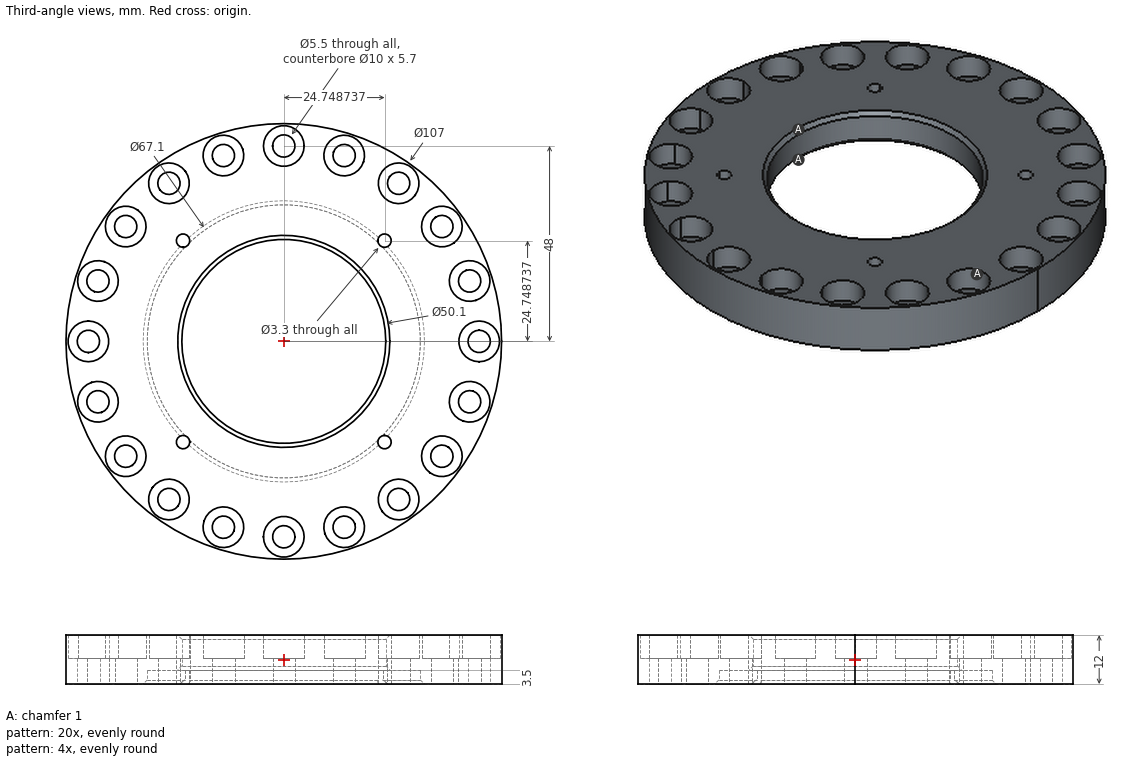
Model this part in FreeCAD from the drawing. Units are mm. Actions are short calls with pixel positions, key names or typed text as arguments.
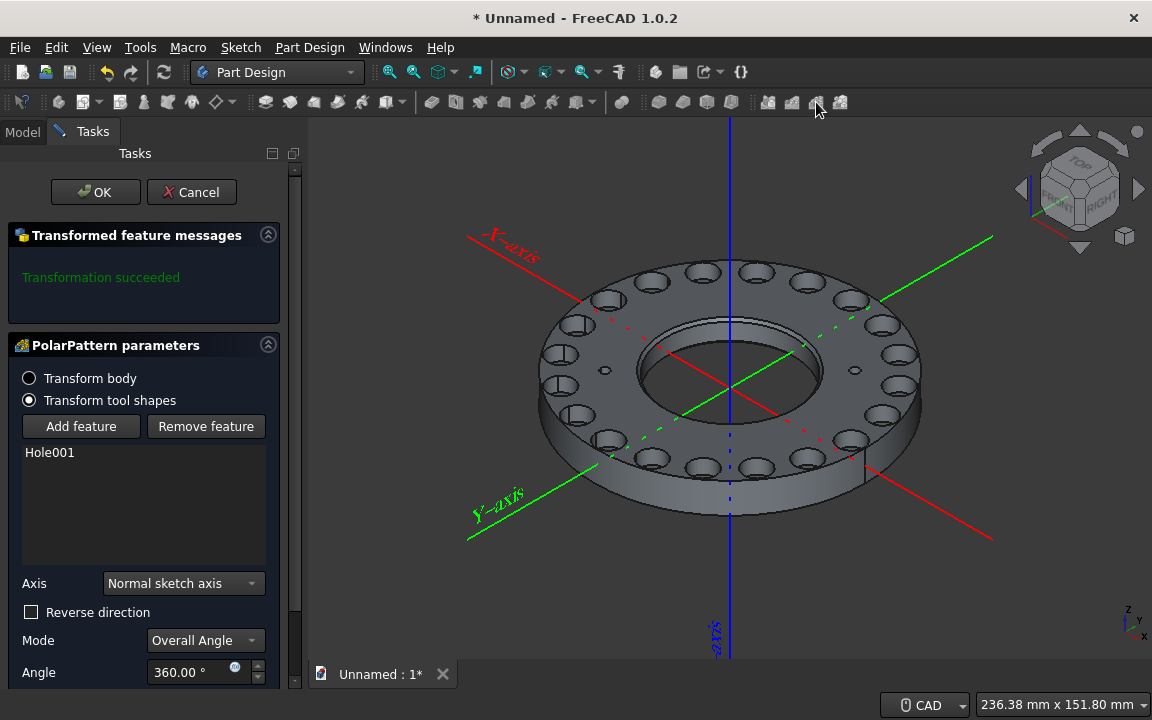
click(184, 584)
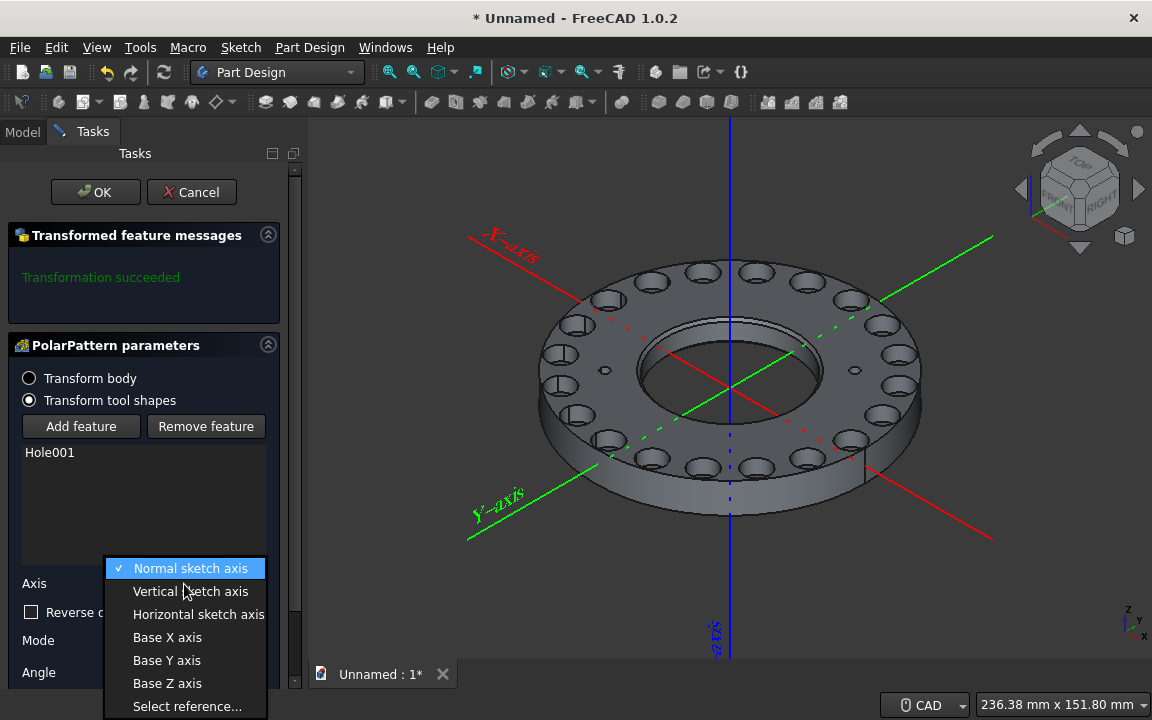
click(184, 684)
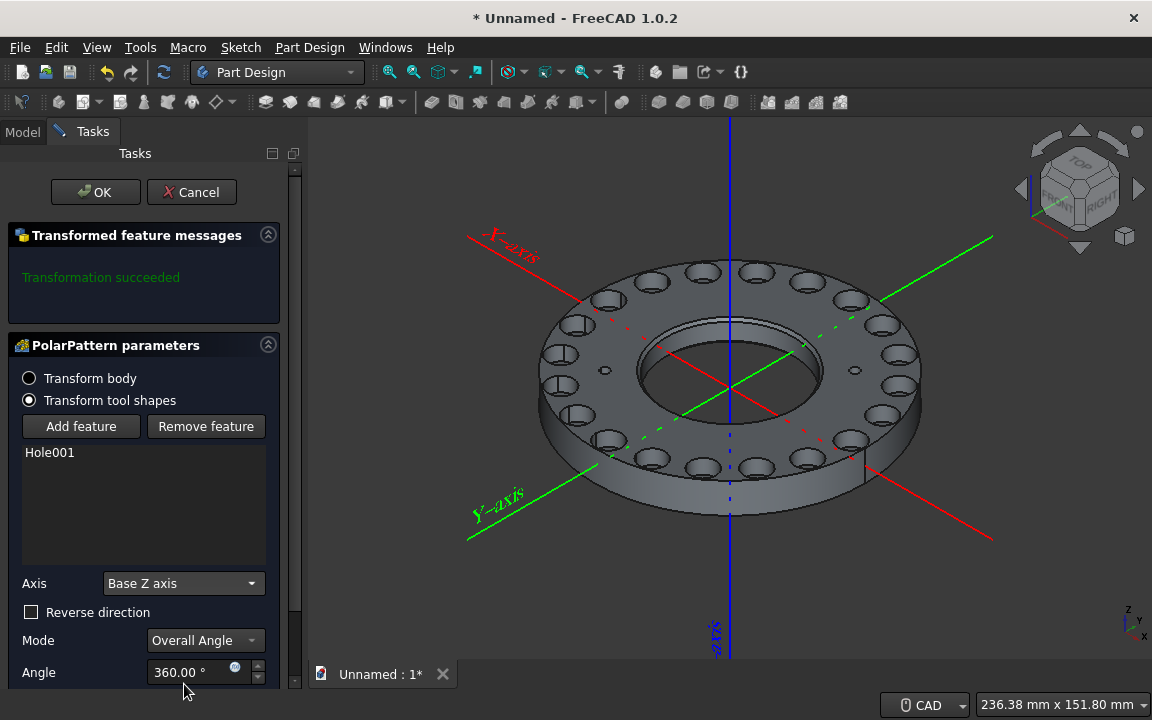
scroll(295, 426, down, 2)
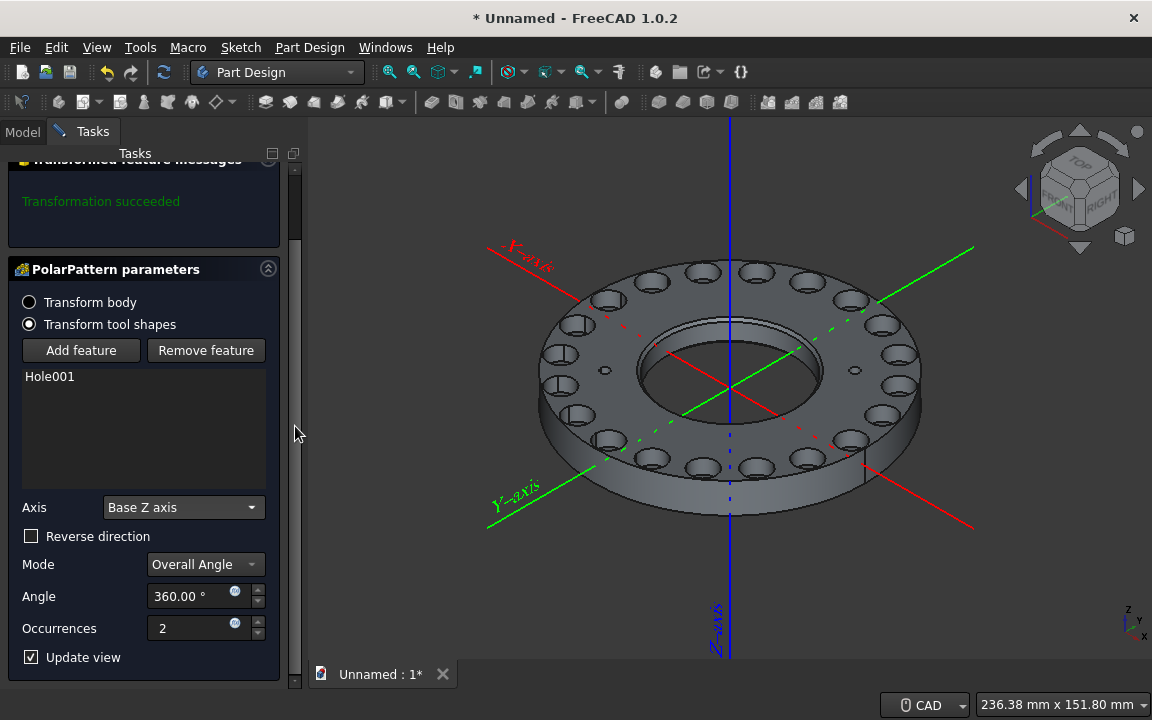
triple_click(198, 628)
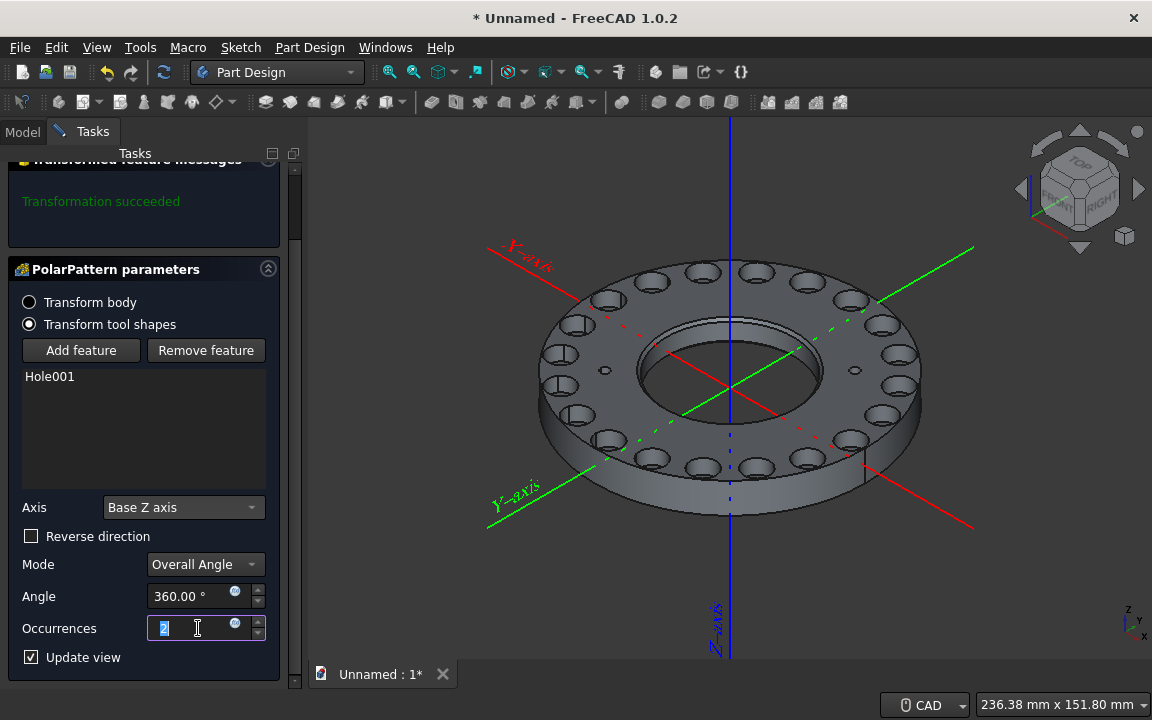
text(4)
key(Tab)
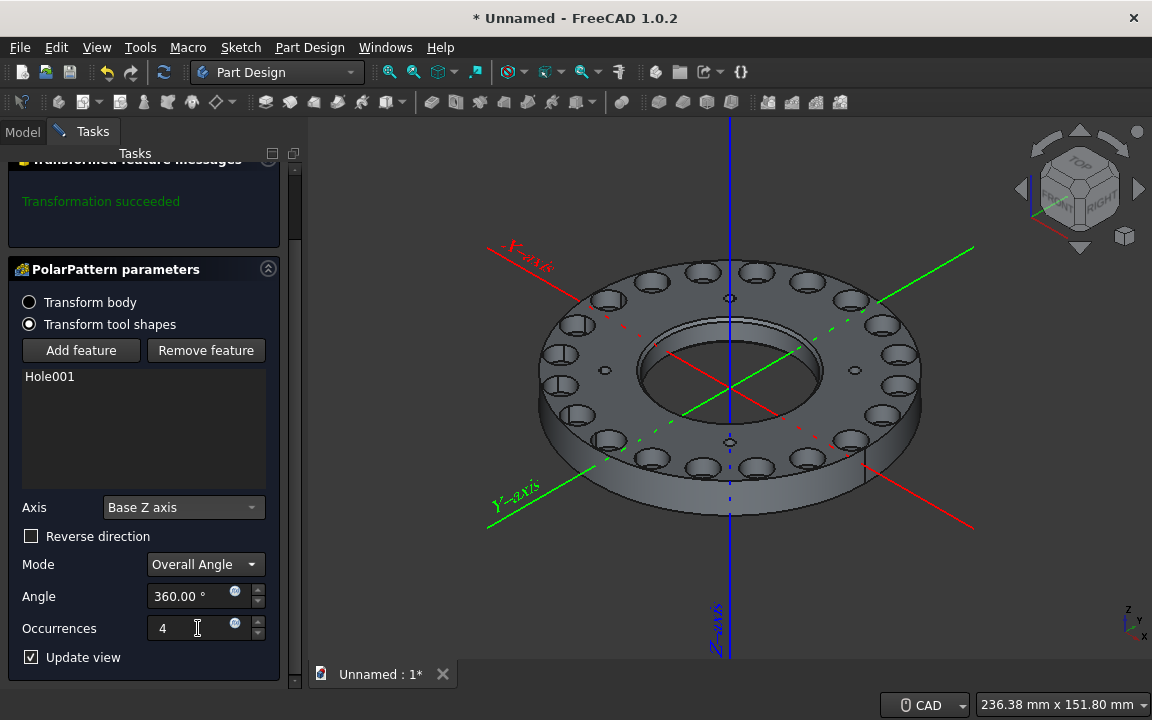
scroll(295, 426, up, 3)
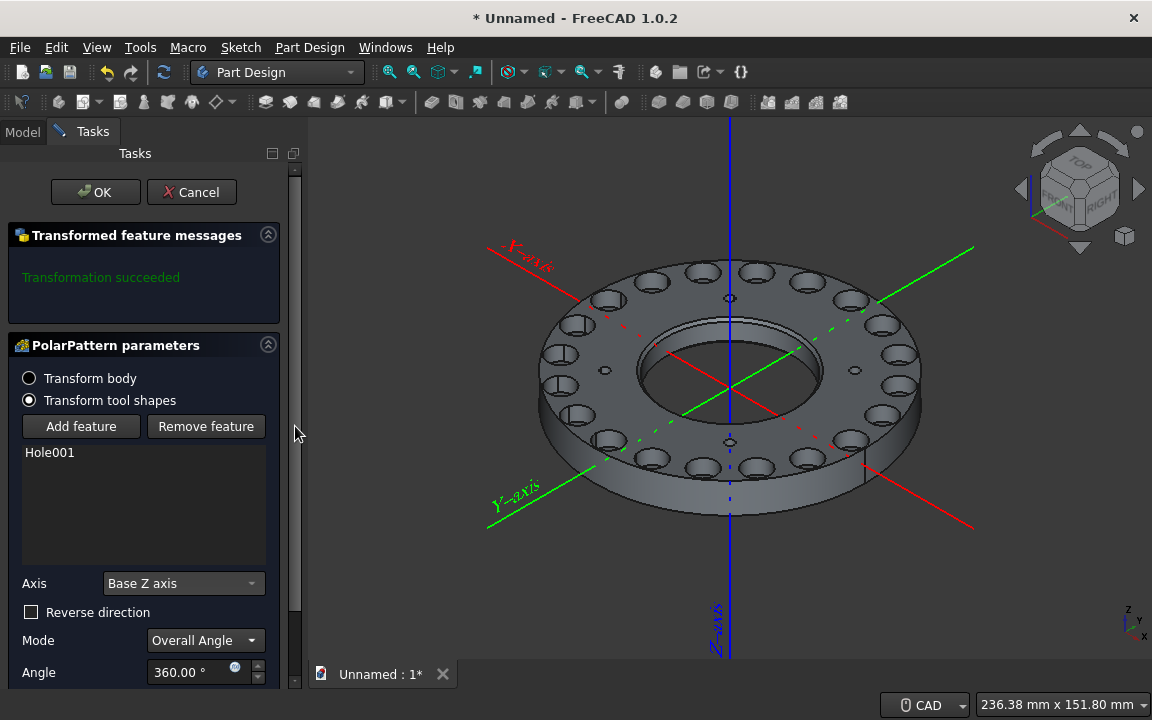
click(96, 192)